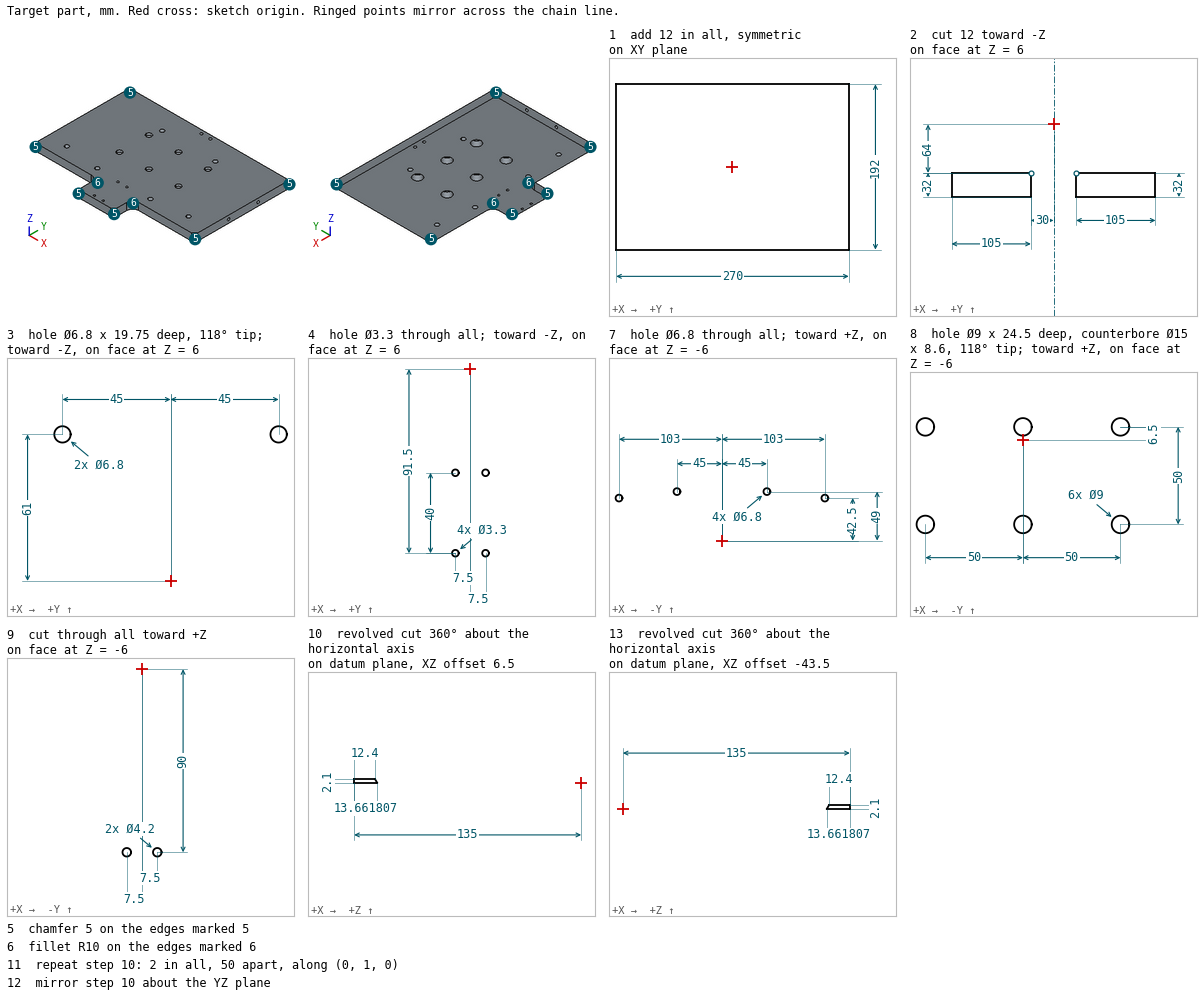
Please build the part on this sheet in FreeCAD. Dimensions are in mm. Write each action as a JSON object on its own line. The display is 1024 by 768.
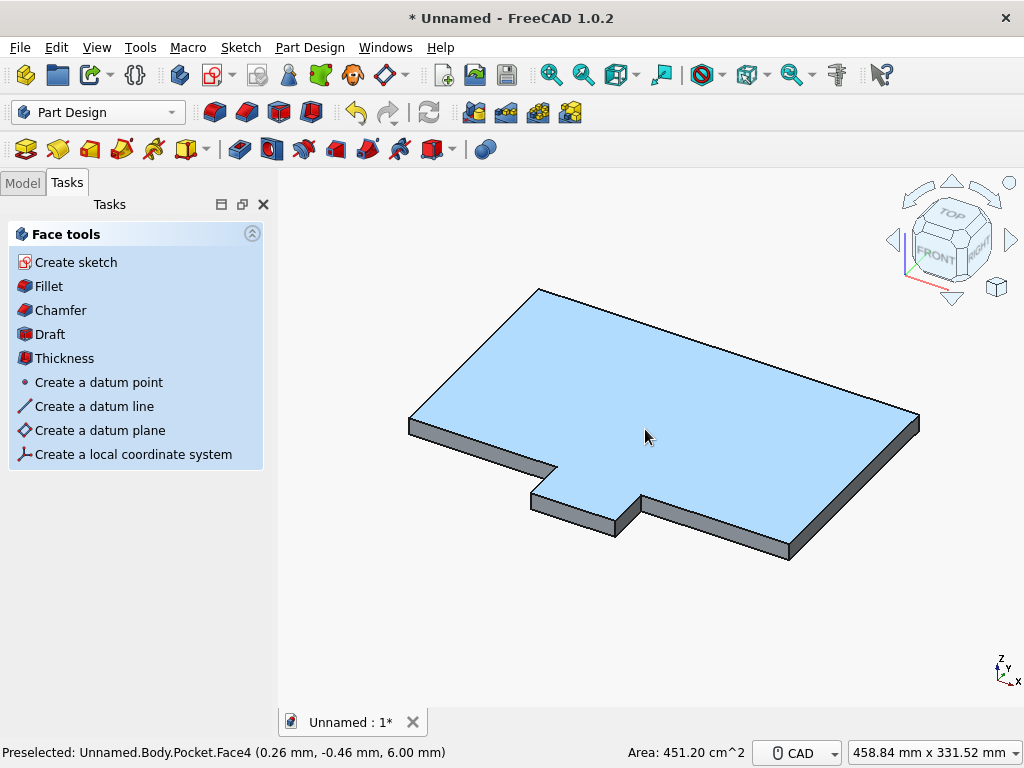
{"action": "left_click", "coordinate": [212, 76]}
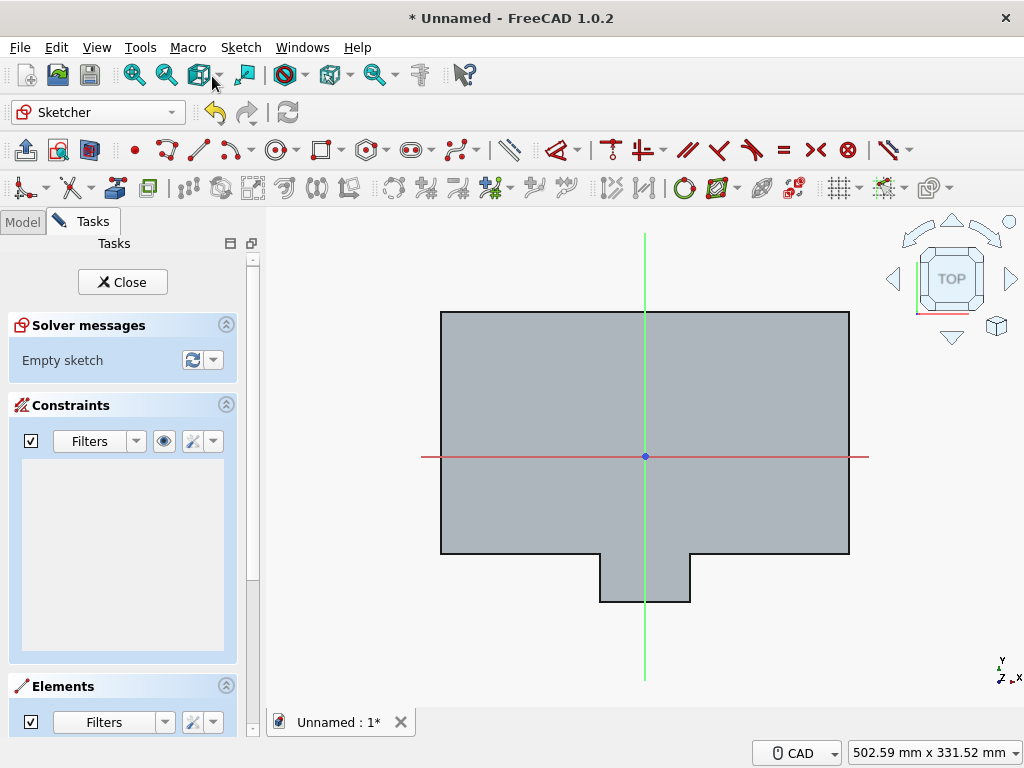
{"action": "scroll", "coordinate": [685, 380], "scroll_direction": "up", "scroll_amount": 5}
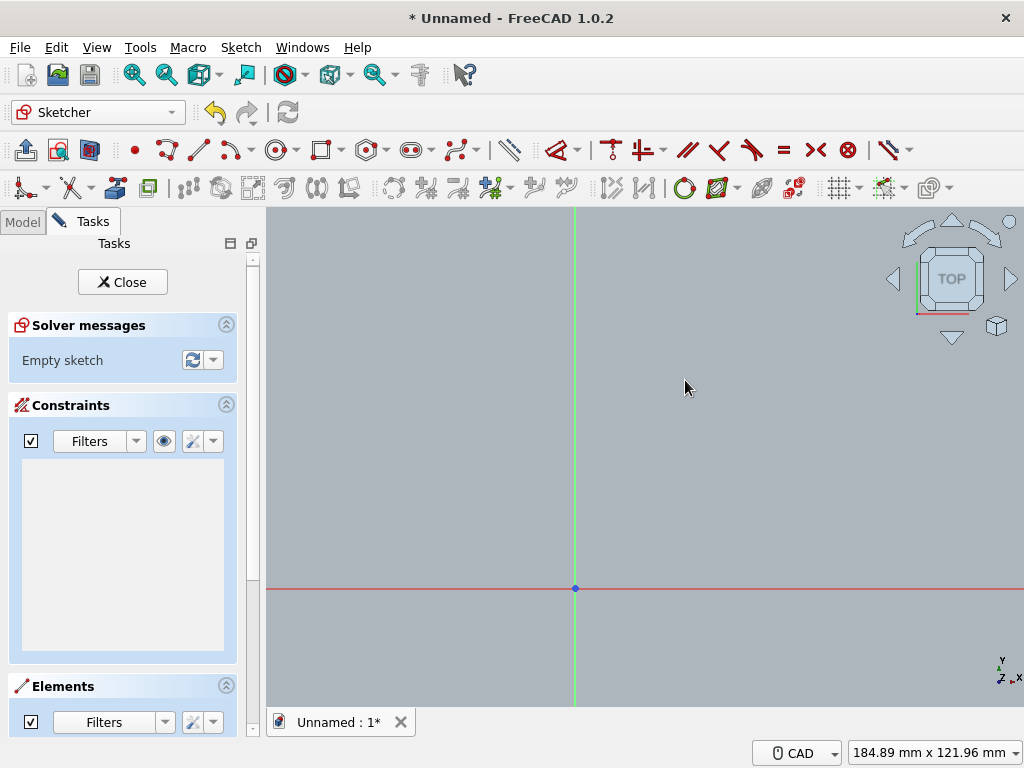
{"action": "key", "text": "g c"}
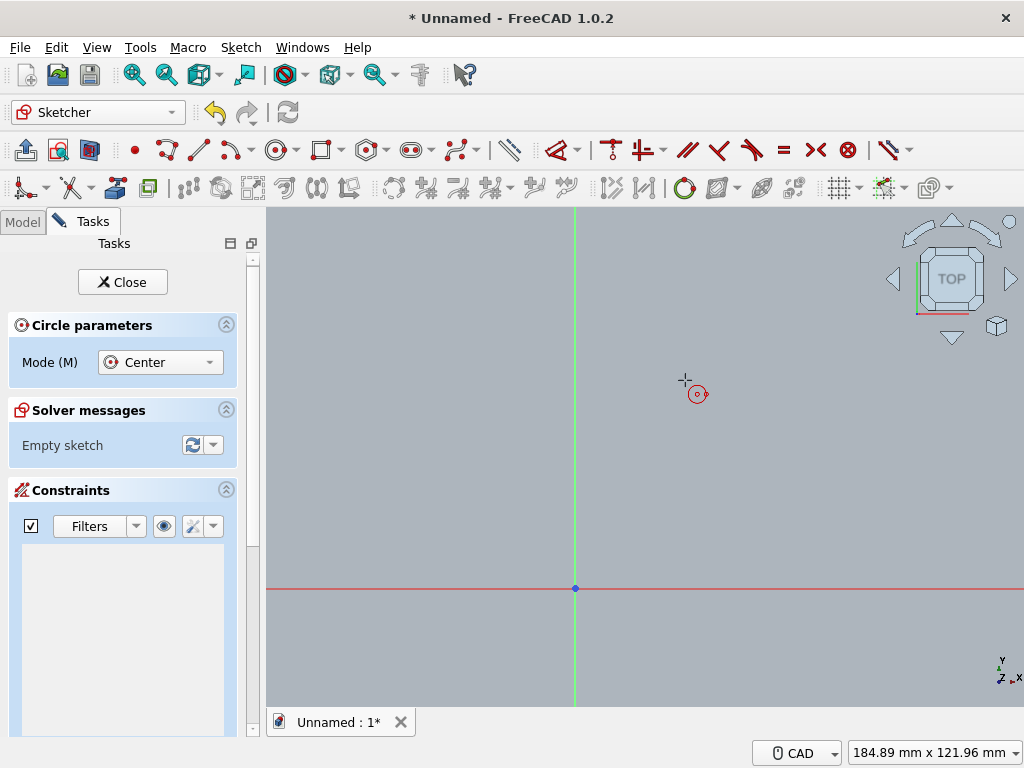
{"action": "scroll", "coordinate": [391, 339], "scroll_direction": "up", "scroll_amount": 3}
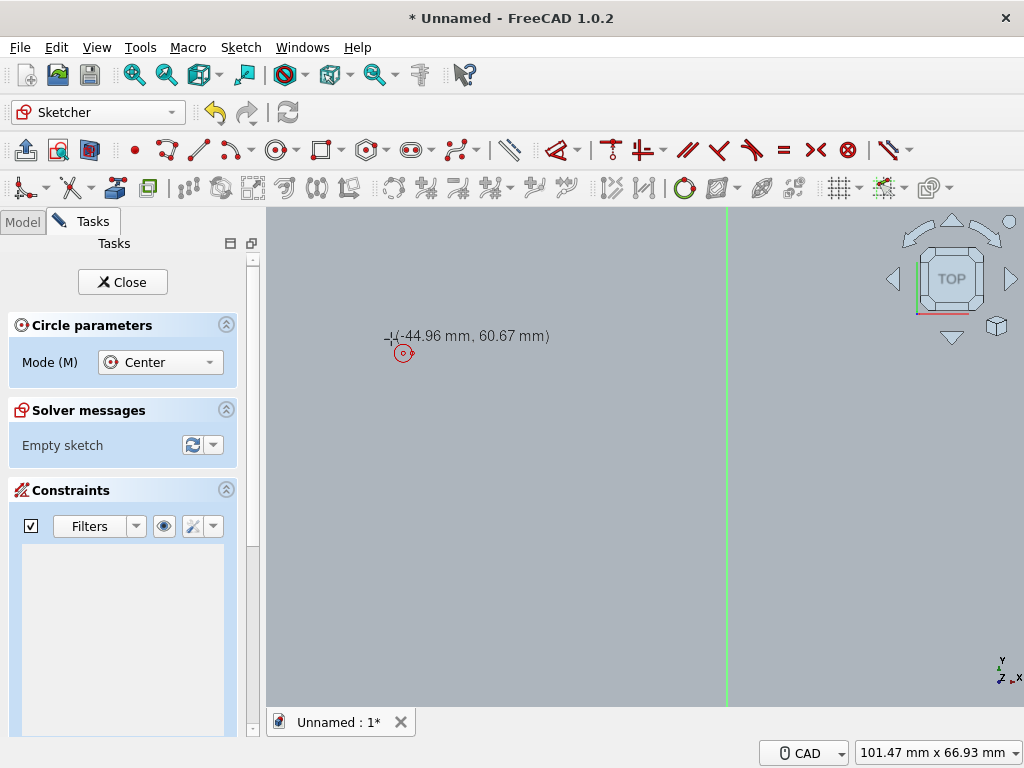
{"action": "left_click", "coordinate": [391, 338]}
{"action": "mouse_move", "coordinate": [409, 320]}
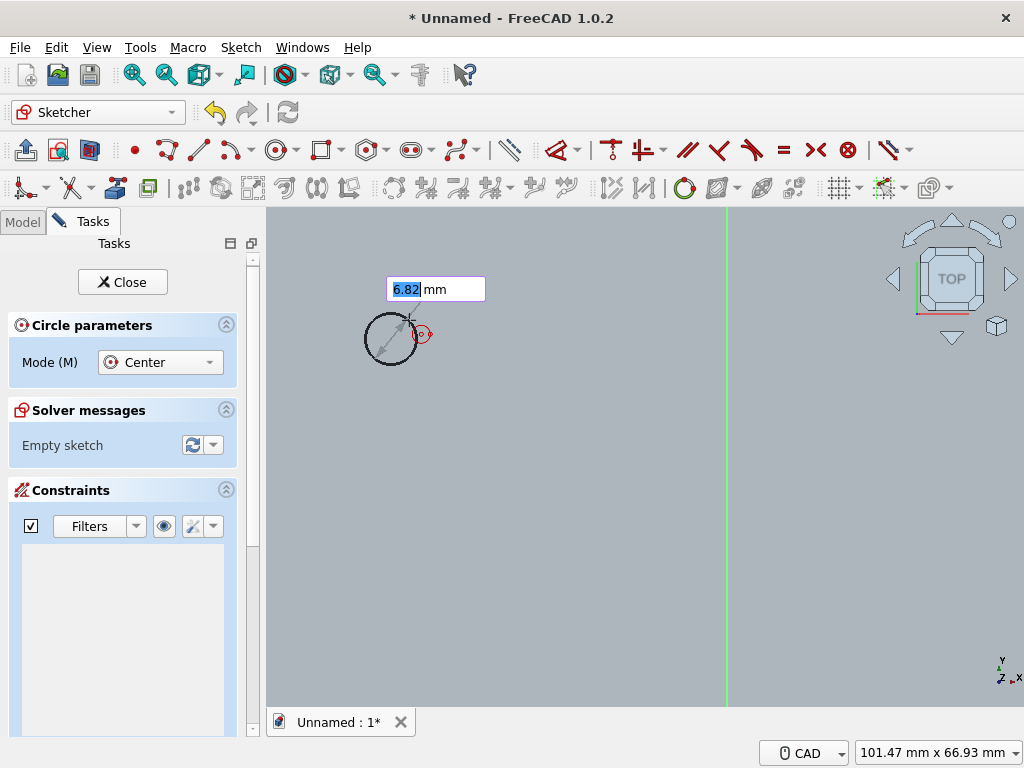
{"action": "type", "text": "6.8"}
{"action": "key", "text": "Return"}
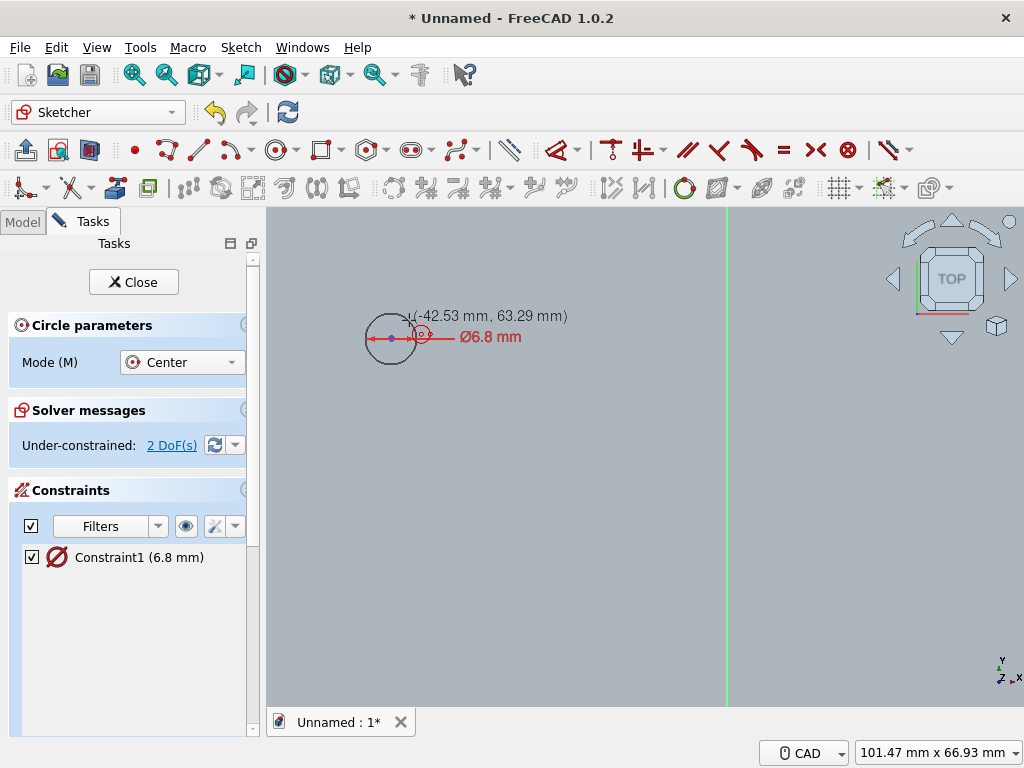
{"action": "scroll", "coordinate": [394, 340], "scroll_direction": "down", "scroll_amount": 3}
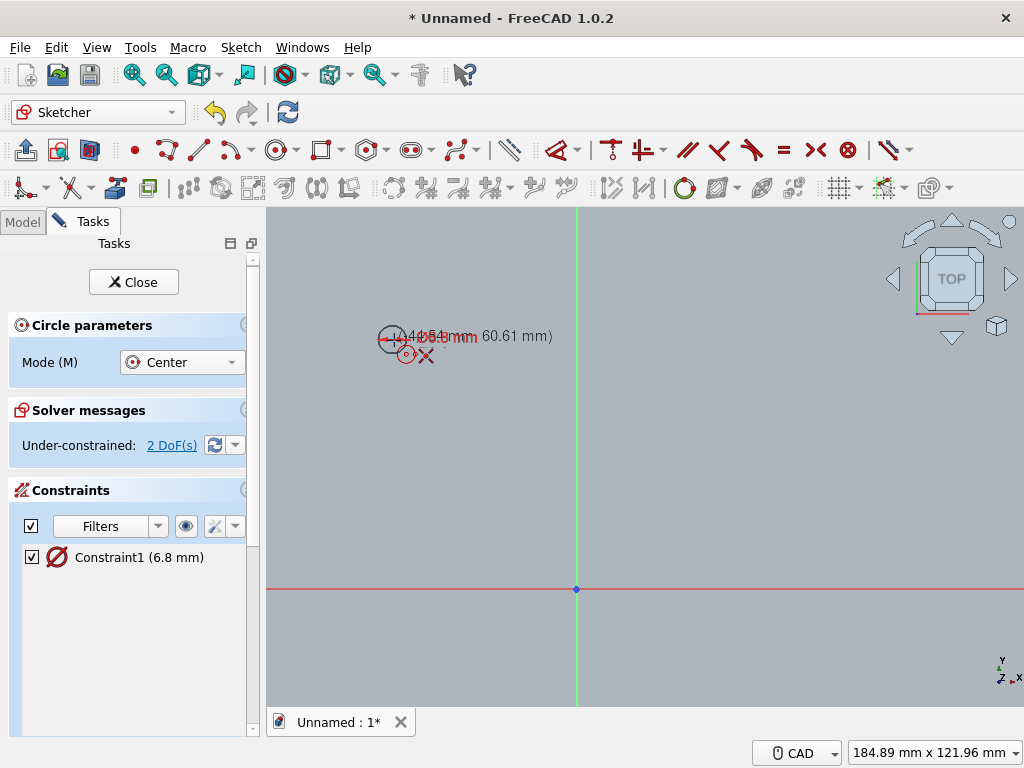
{"action": "scroll", "coordinate": [761, 339], "scroll_direction": "up", "scroll_amount": 3}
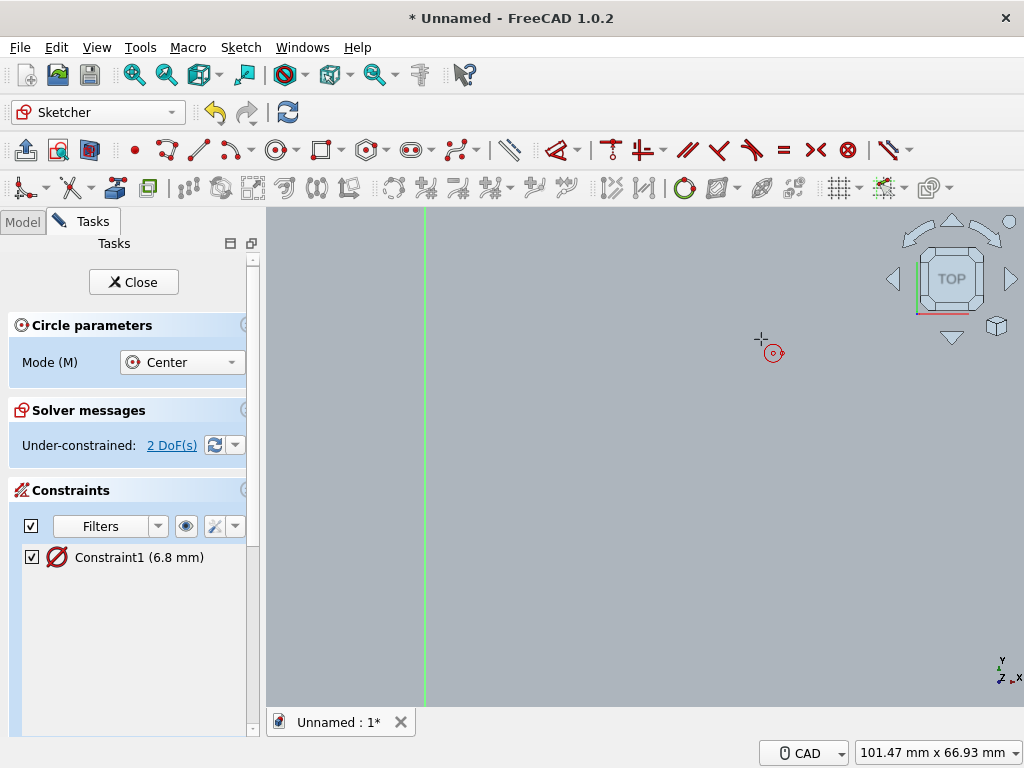
{"action": "left_click", "coordinate": [761, 339]}
{"action": "mouse_move", "coordinate": [779, 321]}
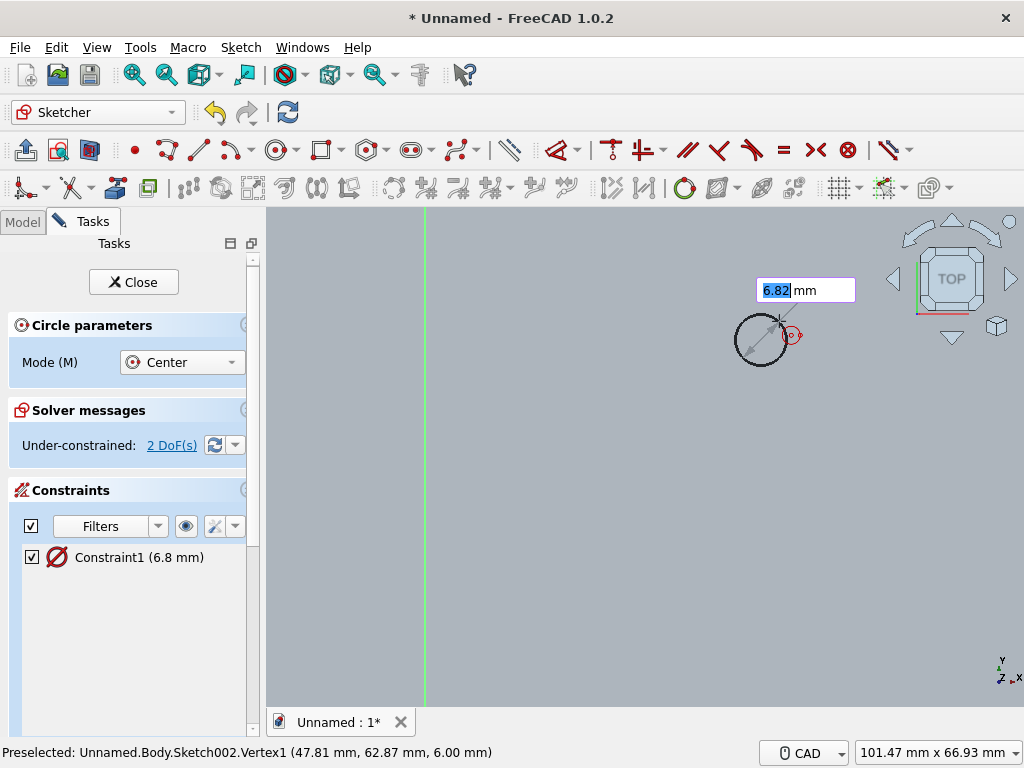
{"action": "type", "text": "6.8"}
{"action": "key", "text": "Return"}
{"action": "key", "text": "Escape"}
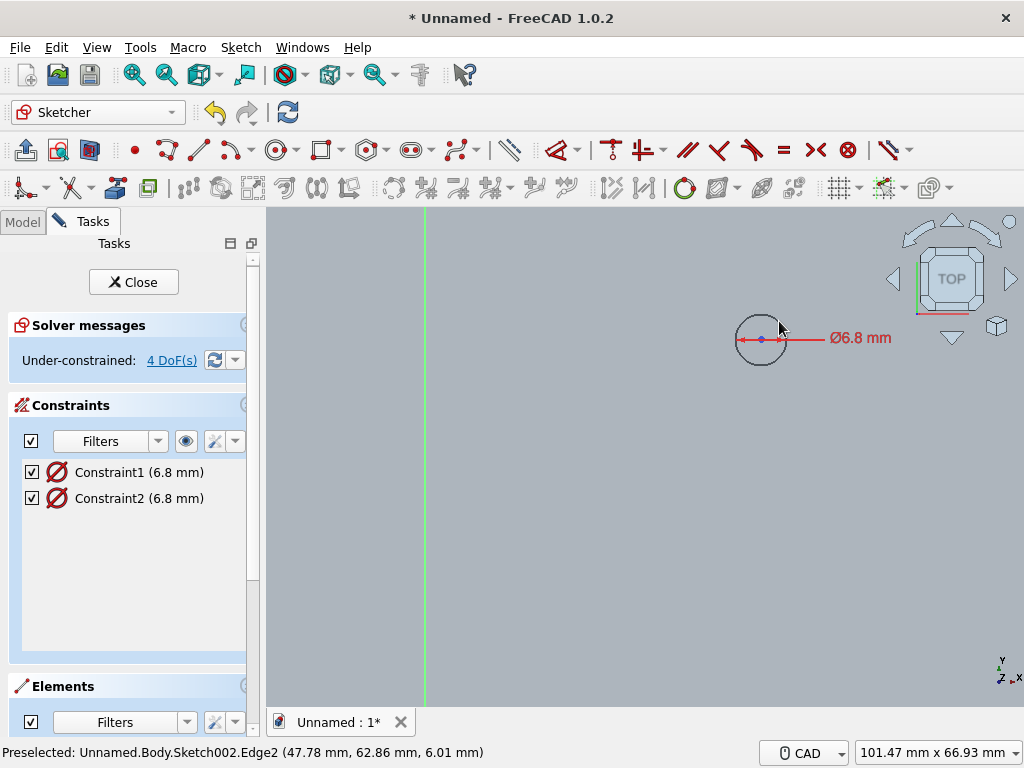
{"action": "scroll", "coordinate": [761, 339], "scroll_direction": "down", "scroll_amount": 3}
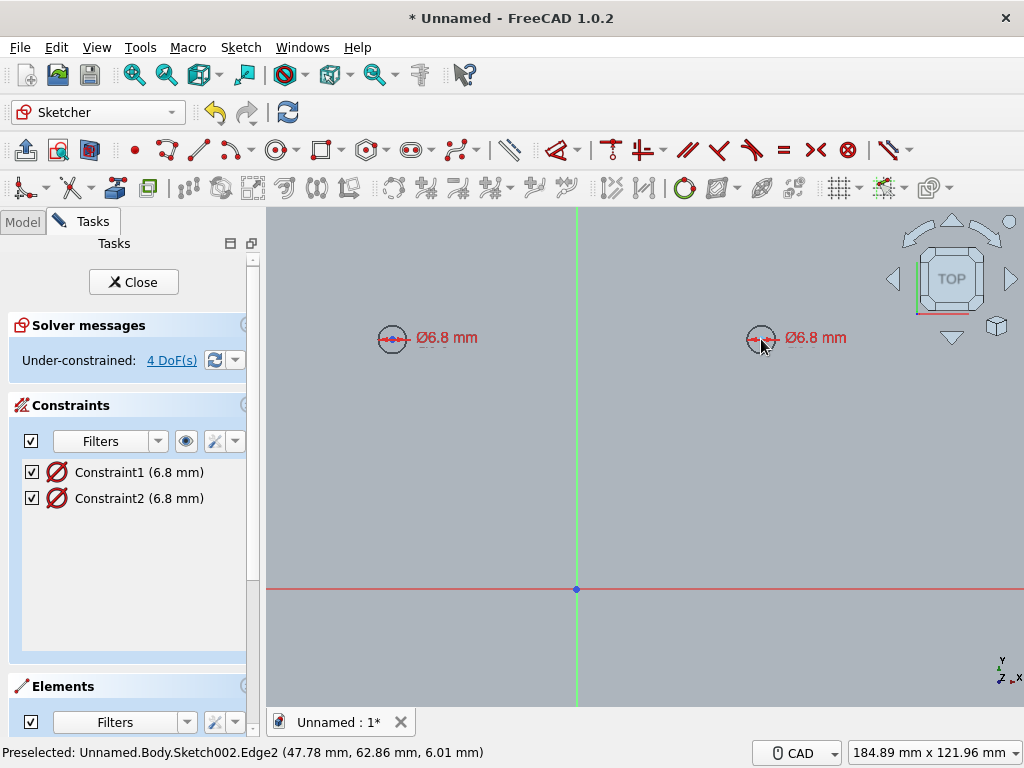
{"action": "left_click", "coordinate": [392, 340]}